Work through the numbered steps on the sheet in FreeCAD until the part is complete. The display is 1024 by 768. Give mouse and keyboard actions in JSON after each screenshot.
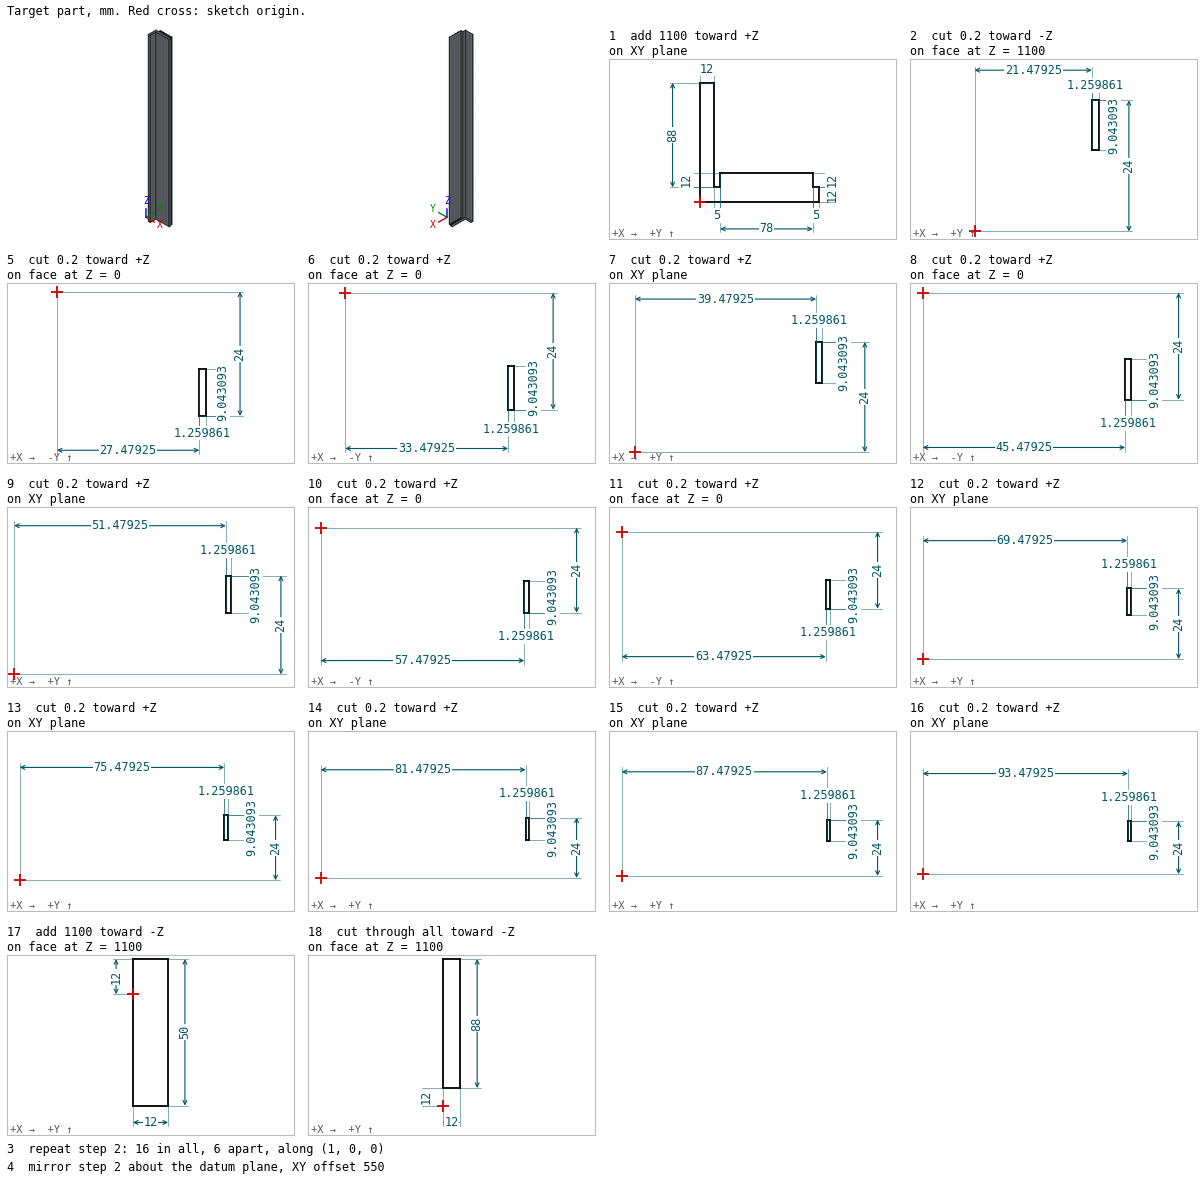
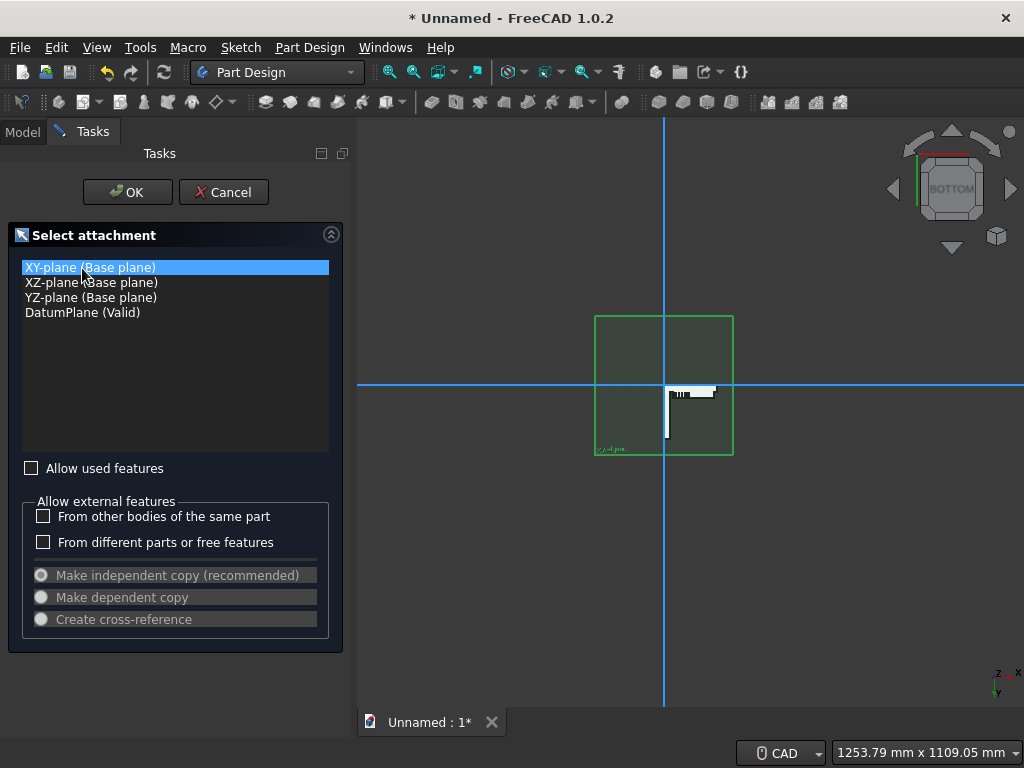
{"action": "left_click", "coordinate": [128, 192]}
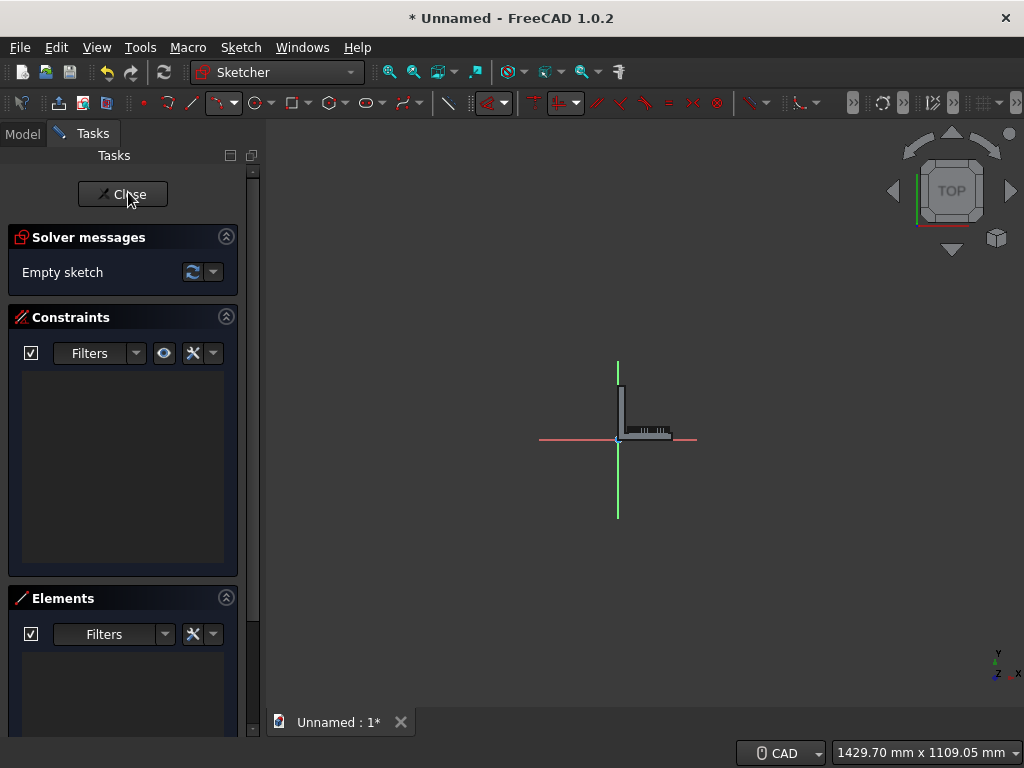
{"action": "left_click", "coordinate": [108, 104]}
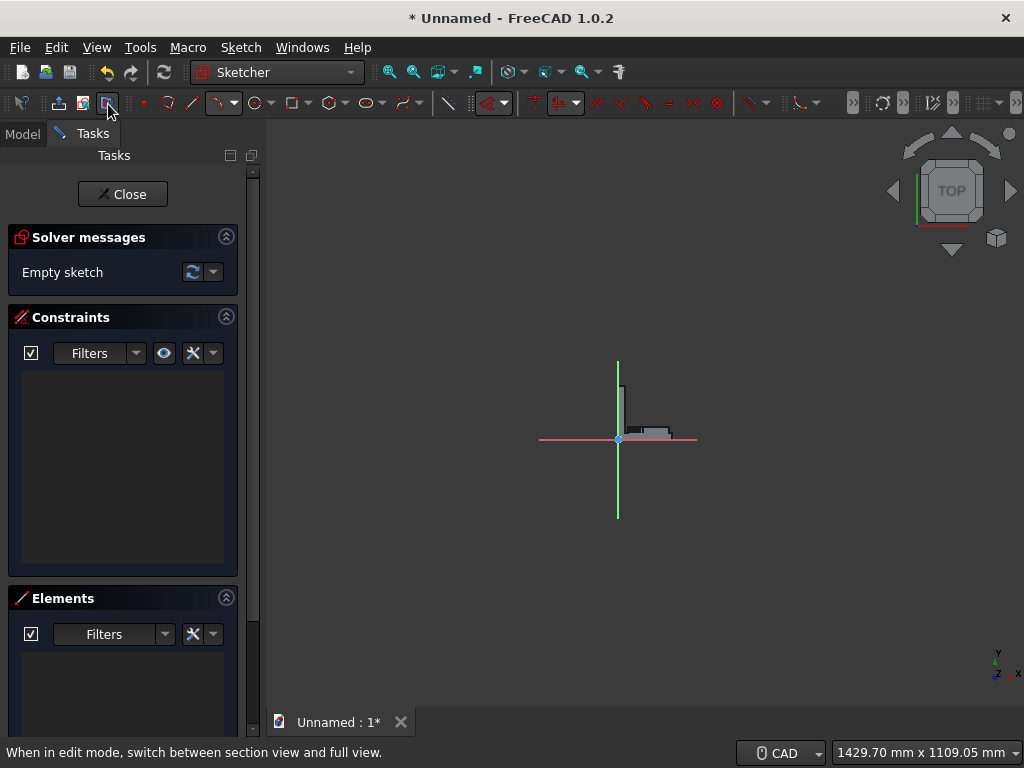
{"action": "scroll", "coordinate": [650, 430], "scroll_direction": "up", "scroll_amount": 15}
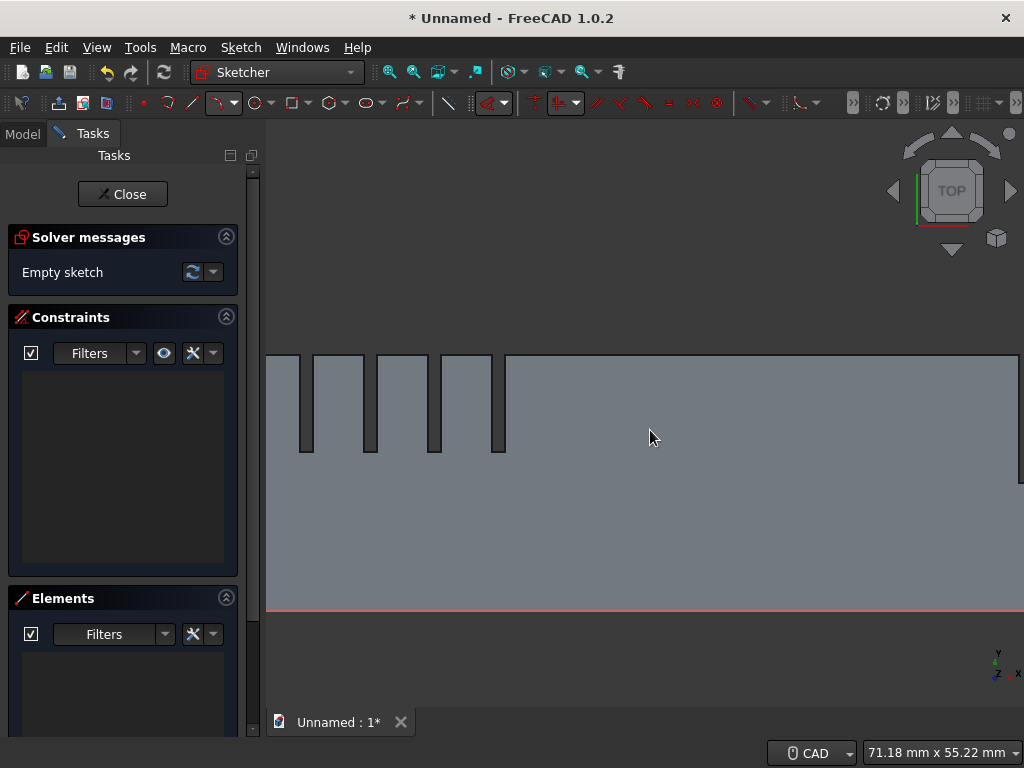
{"action": "scroll", "coordinate": [558, 400], "scroll_direction": "up", "scroll_amount": 7}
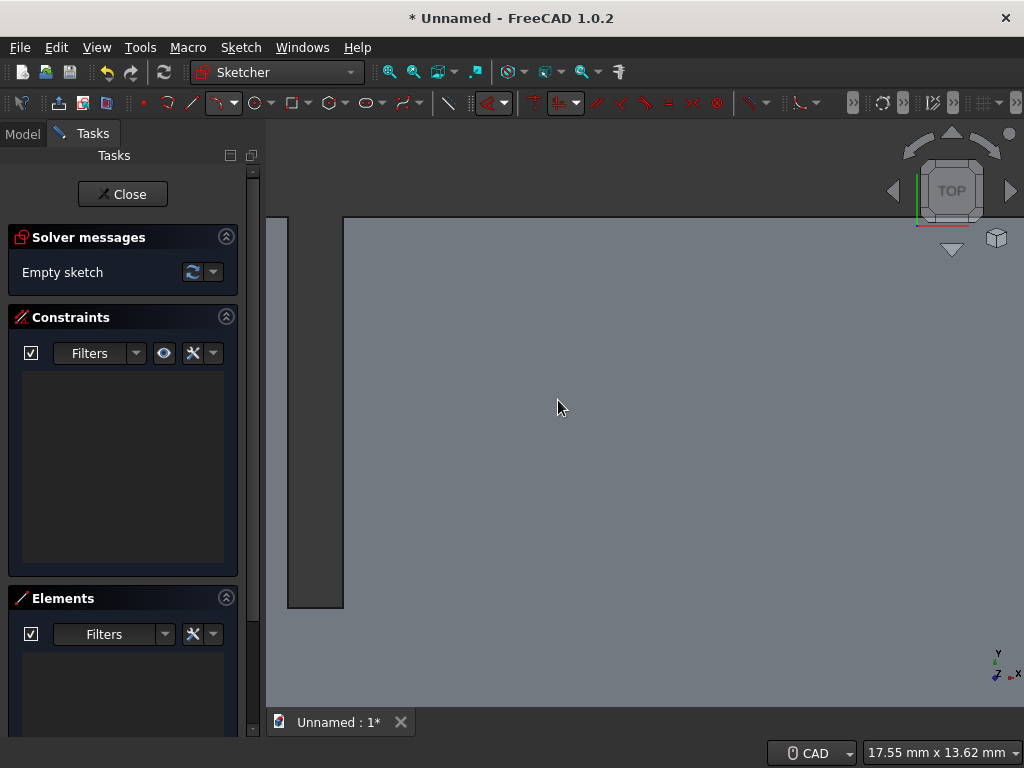
{"action": "left_click", "coordinate": [292, 104]}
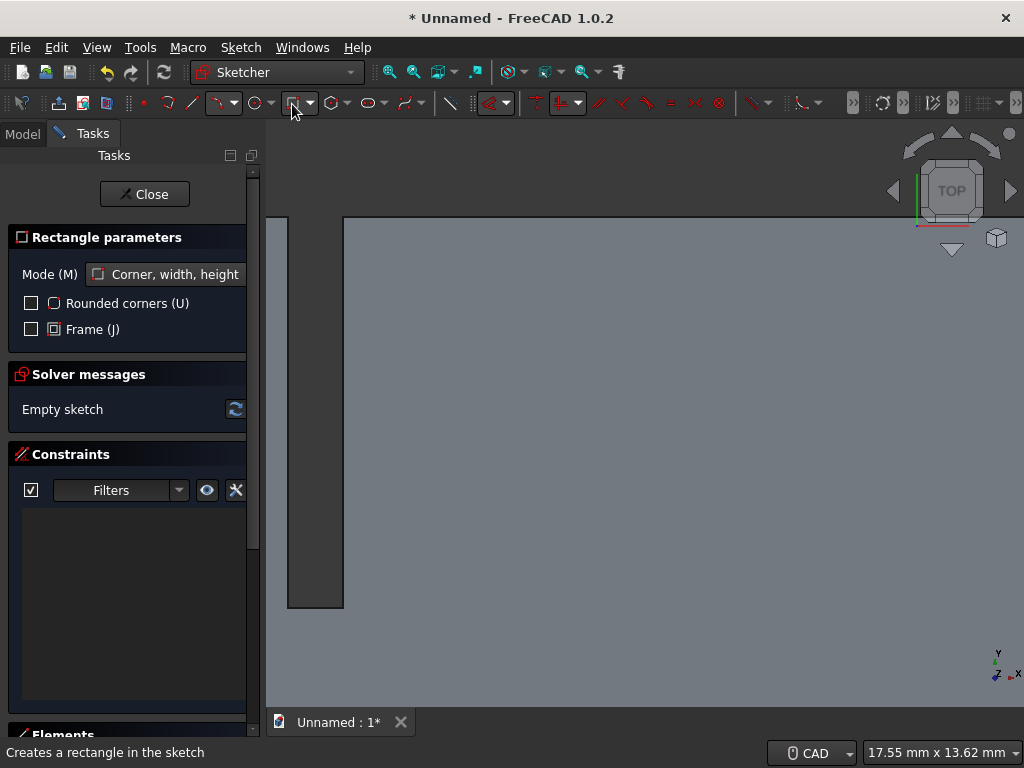
{"action": "left_click", "coordinate": [547, 217]}
{"action": "mouse_move", "coordinate": [602, 608]}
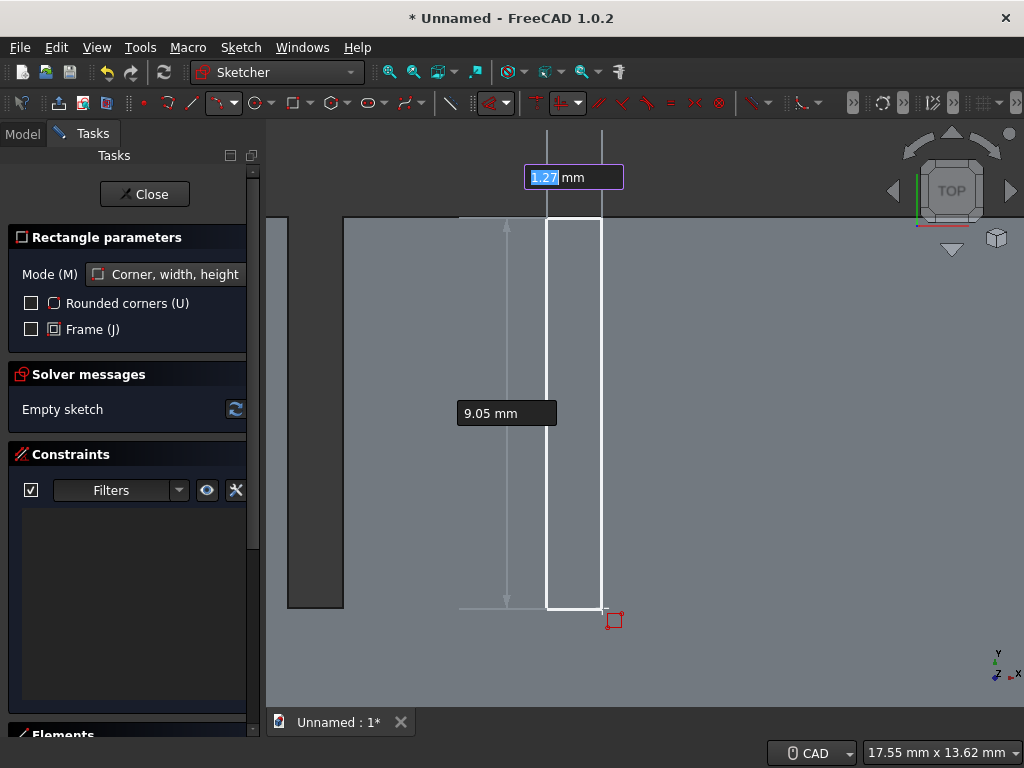
{"action": "type", "text": "1.259861"}
{"action": "key", "text": "Tab"}
{"action": "type", "text": "9.043093"}
{"action": "key", "text": "Return"}
{"action": "key", "text": "Escape"}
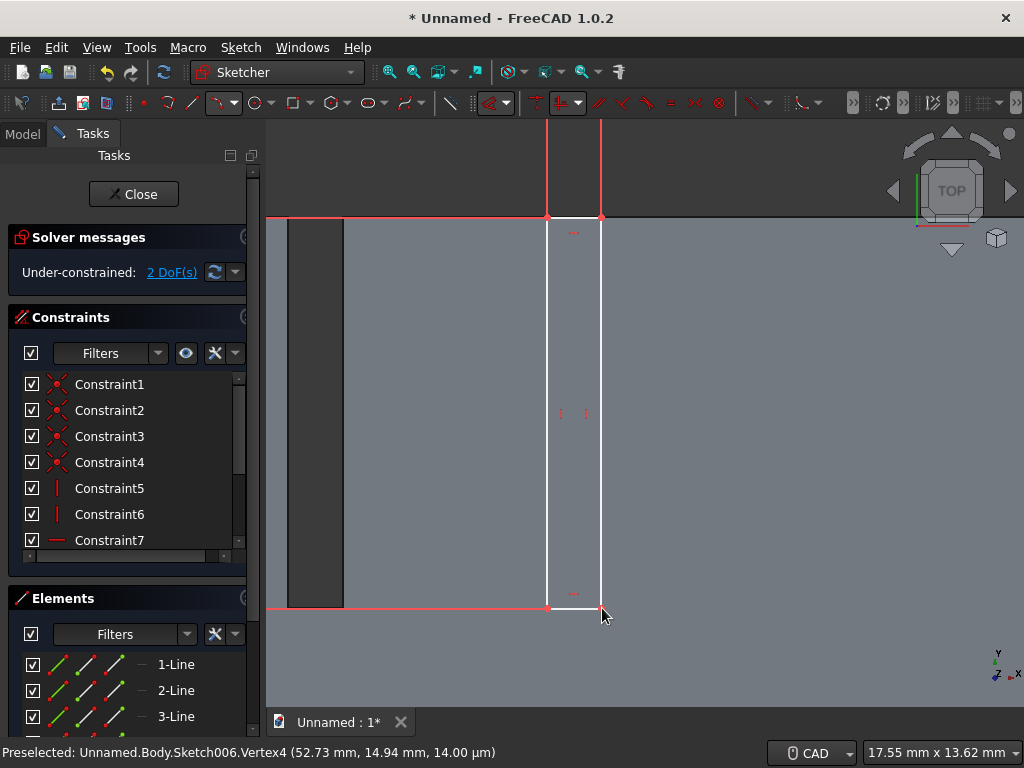
{"action": "left_click", "coordinate": [547, 218]}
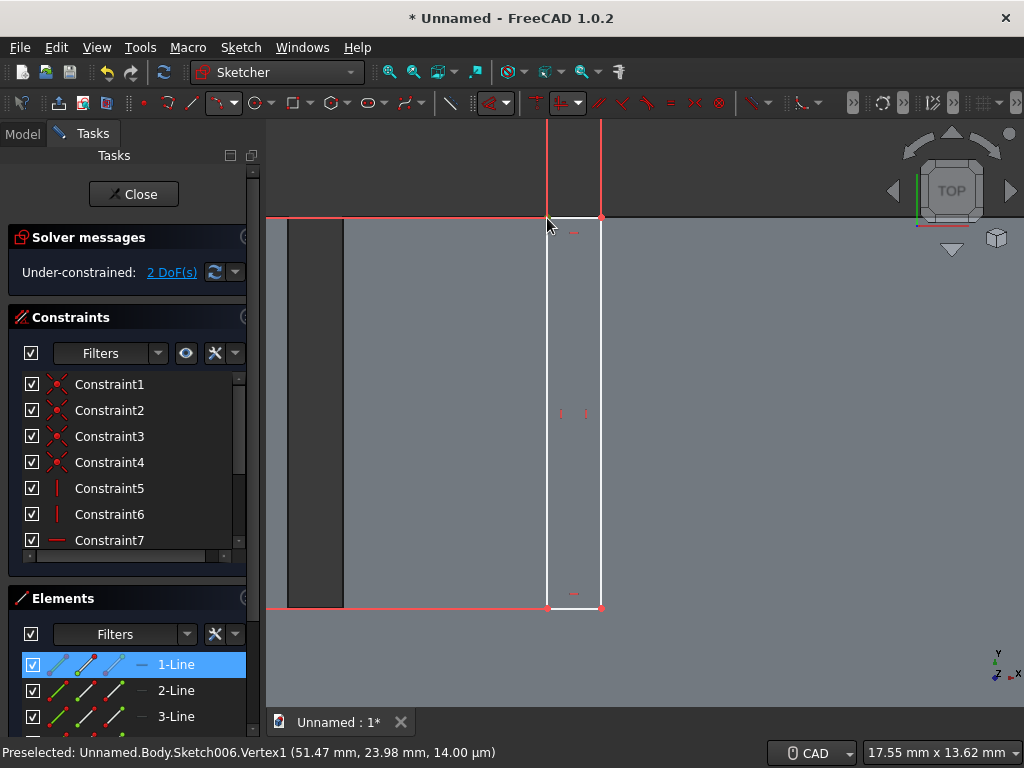
{"action": "key", "text": "i"}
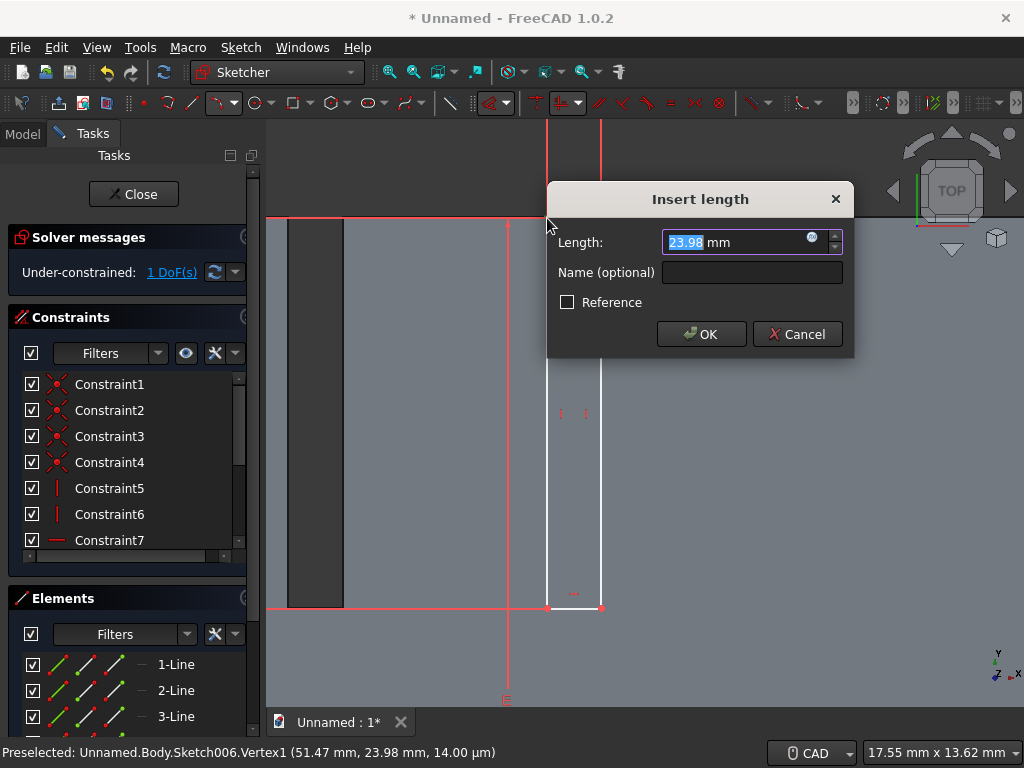
{"action": "type", "text": "24"}
{"action": "key", "text": "Return"}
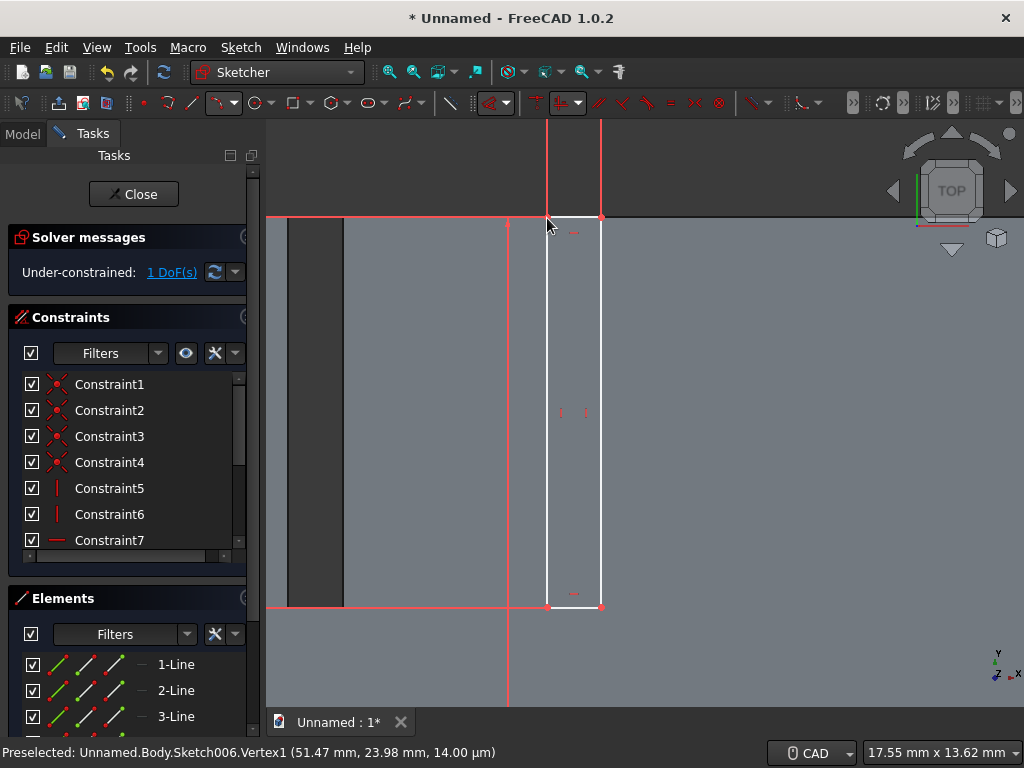
{"action": "left_click", "coordinate": [547, 217]}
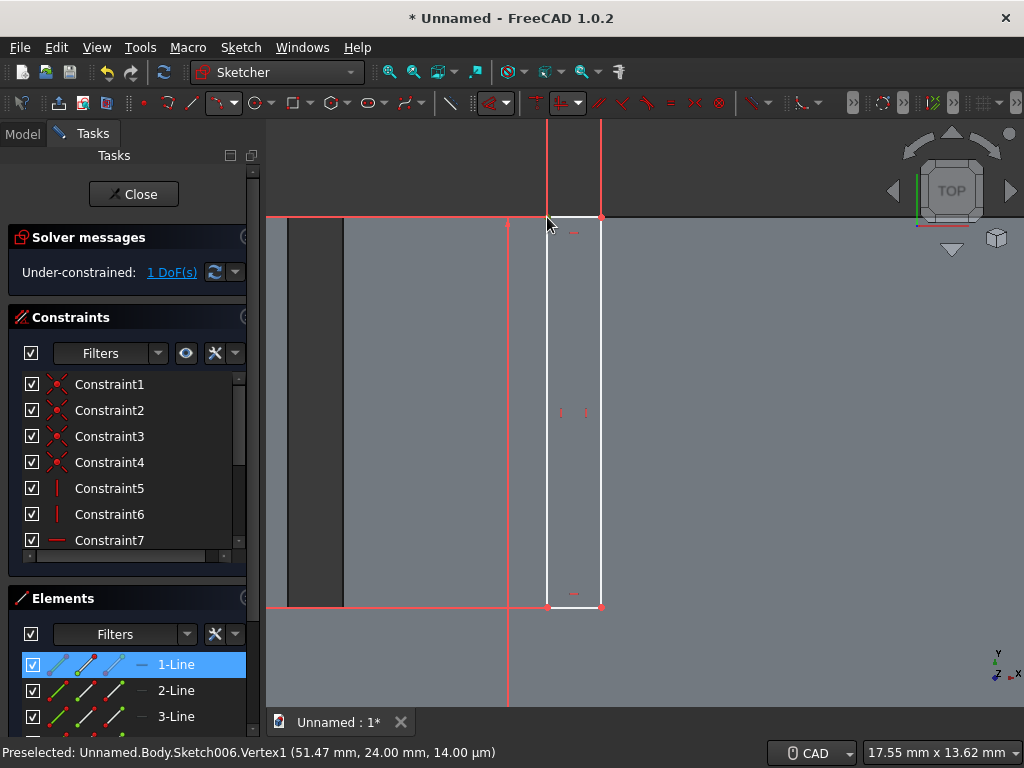
{"action": "left_click", "coordinate": [508, 104]}